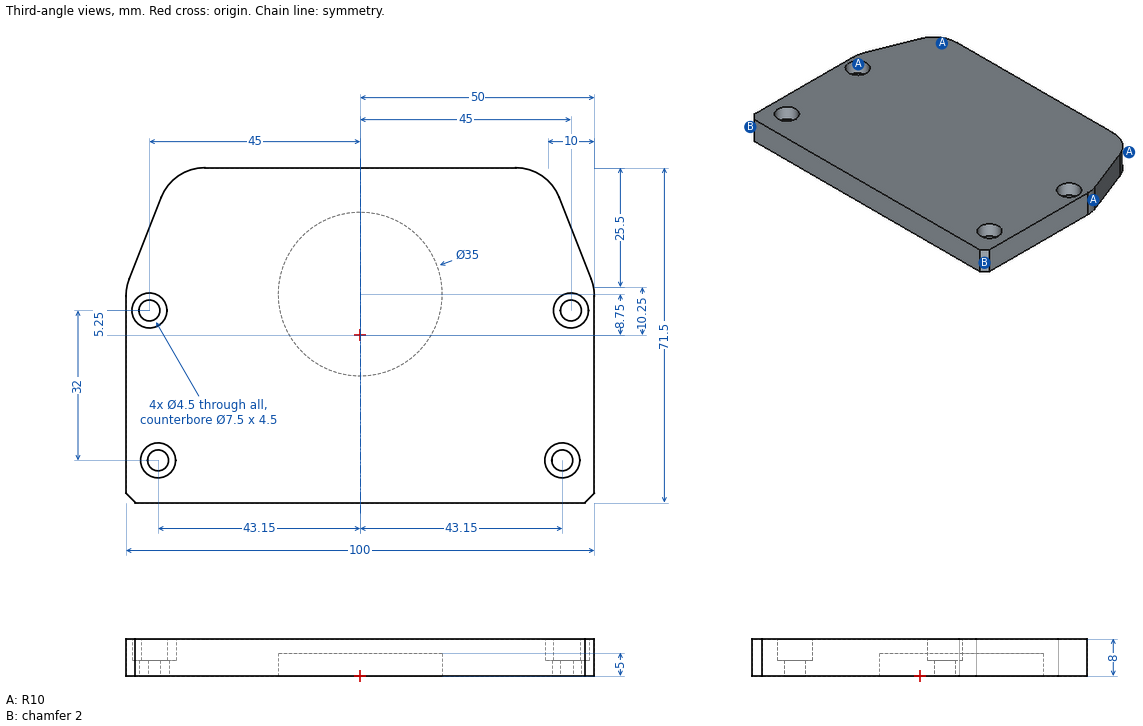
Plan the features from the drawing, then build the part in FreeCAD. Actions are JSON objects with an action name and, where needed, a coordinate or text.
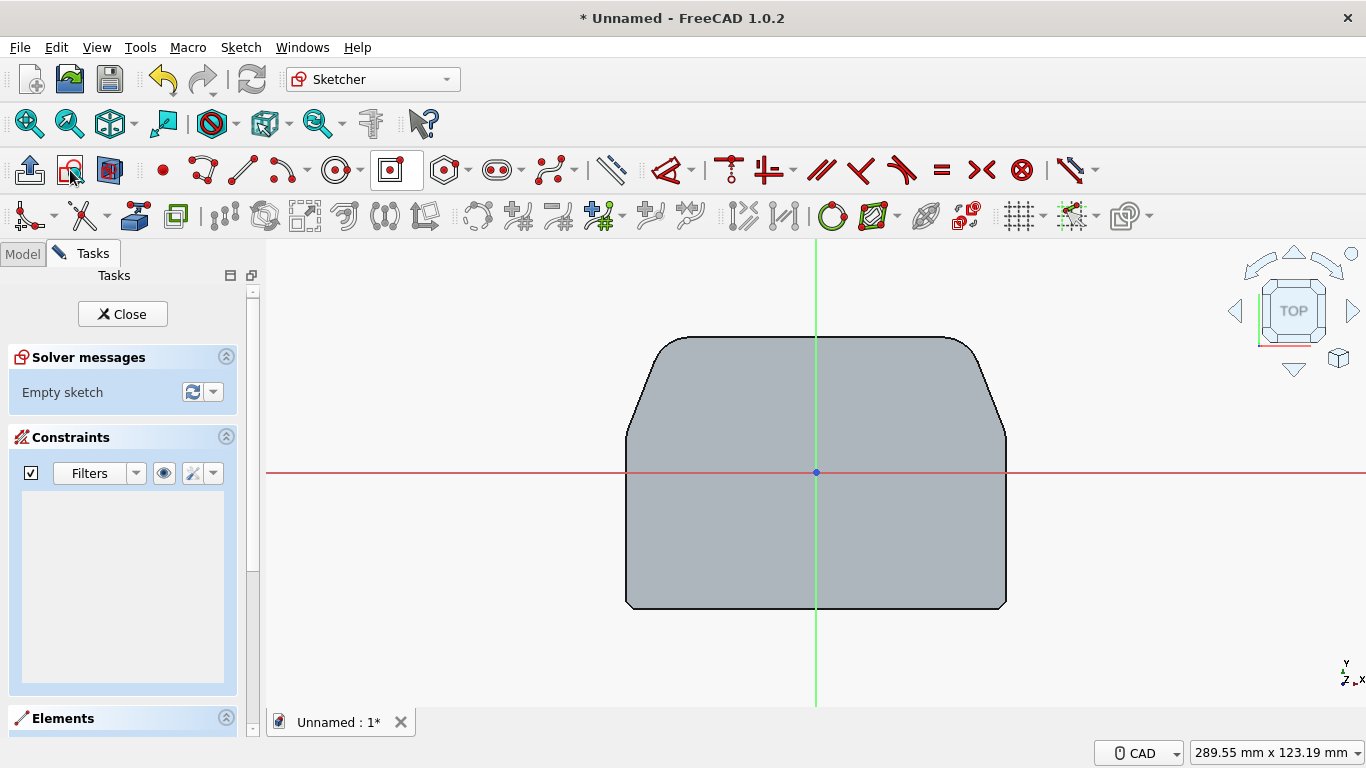
{"action": "scroll", "coordinate": [899, 564], "scroll_direction": "up", "scroll_amount": 3}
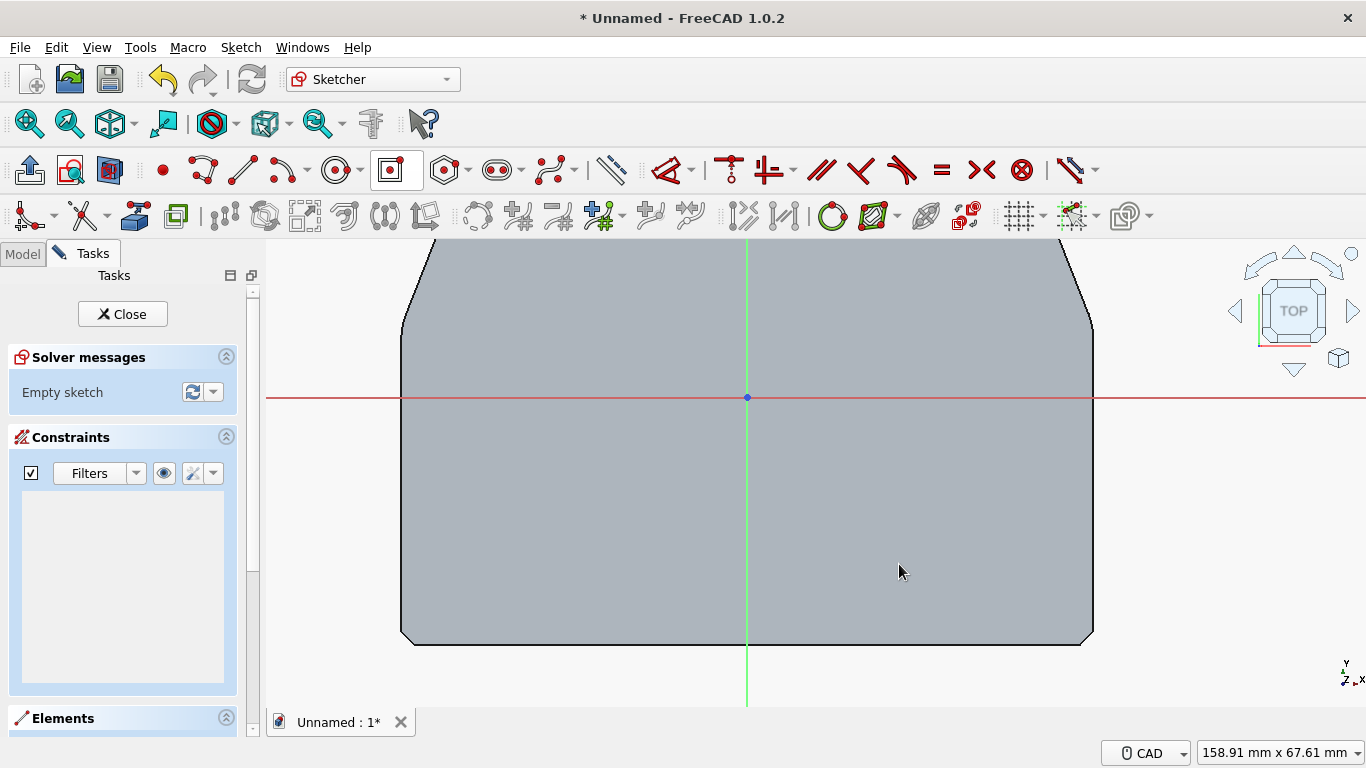
{"action": "left_click", "coordinate": [336, 170]}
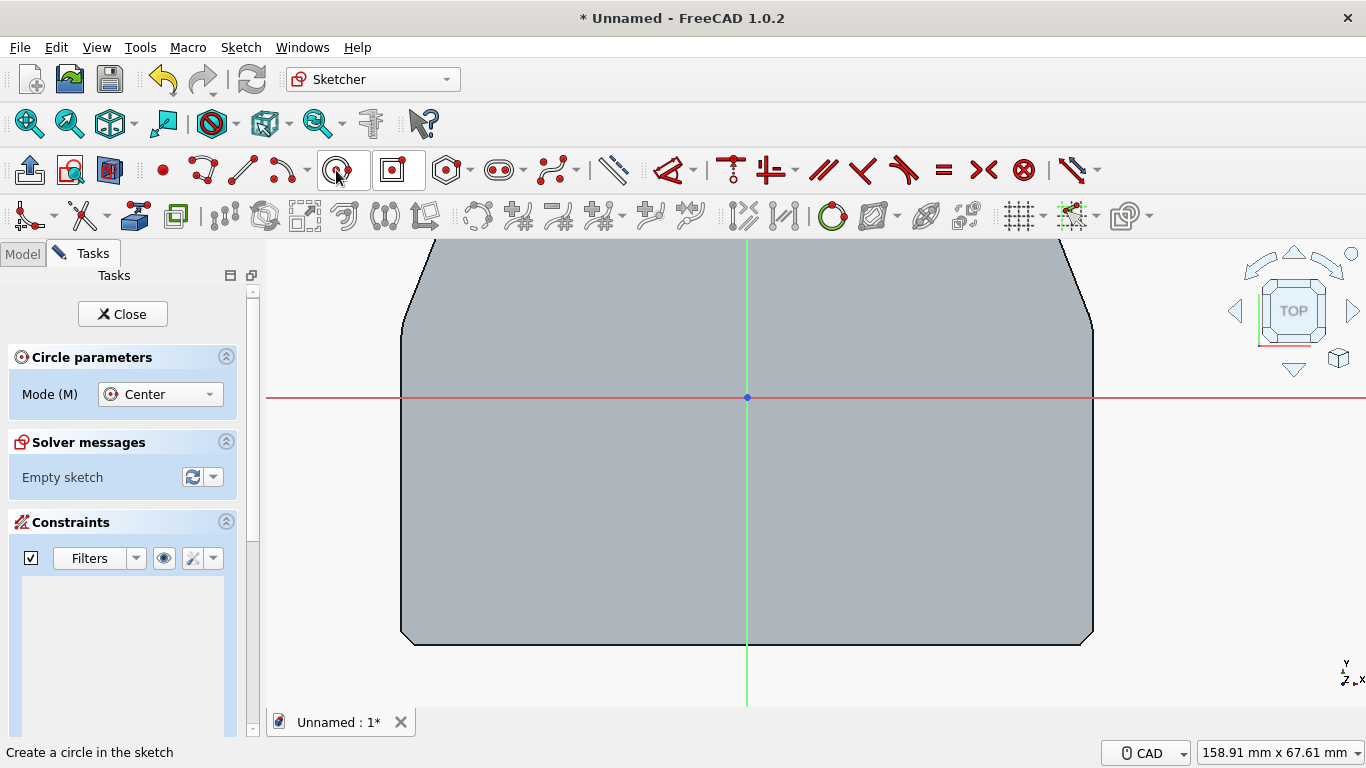
{"action": "scroll", "coordinate": [436, 361], "scroll_direction": "up", "scroll_amount": 2}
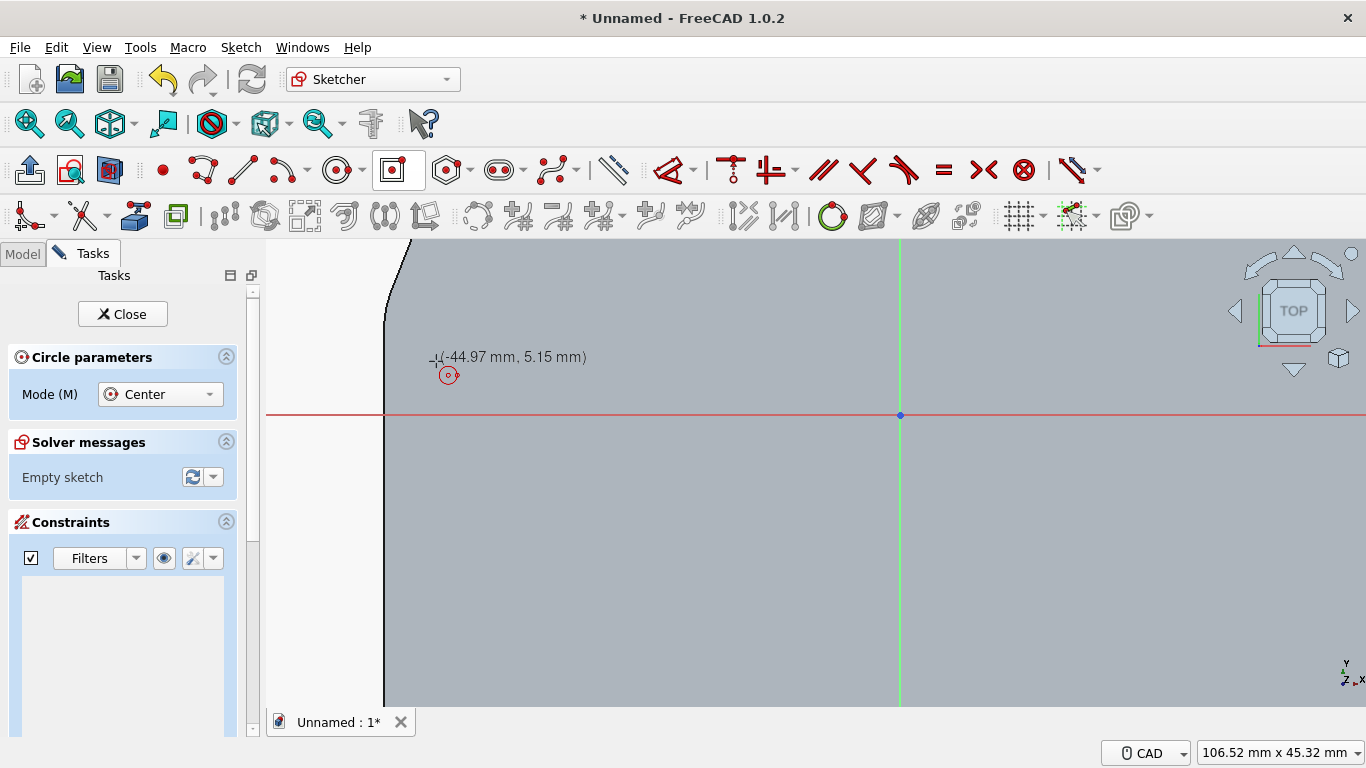
{"action": "left_click", "coordinate": [436, 361]}
{"action": "left_click", "coordinate": [452, 345]}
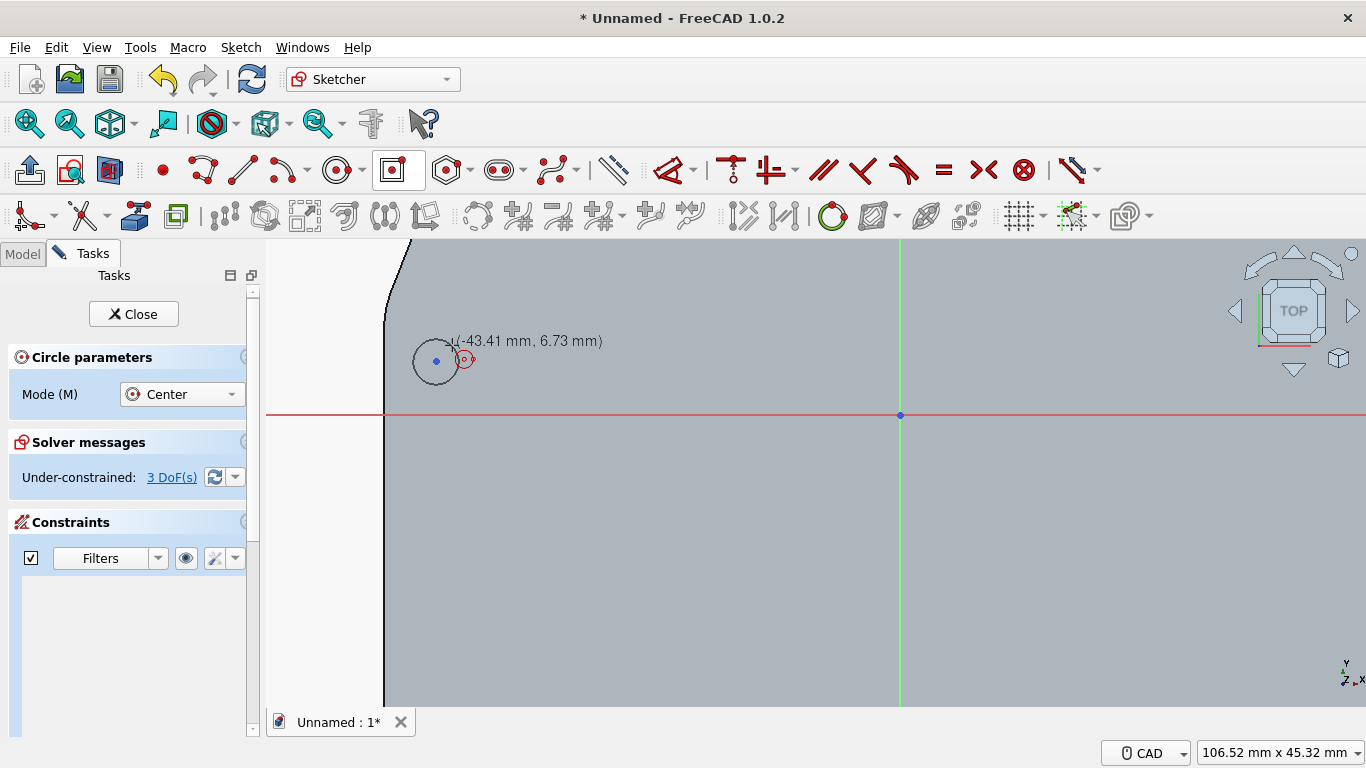
{"action": "scroll", "coordinate": [437, 364], "scroll_direction": "down", "scroll_amount": 2}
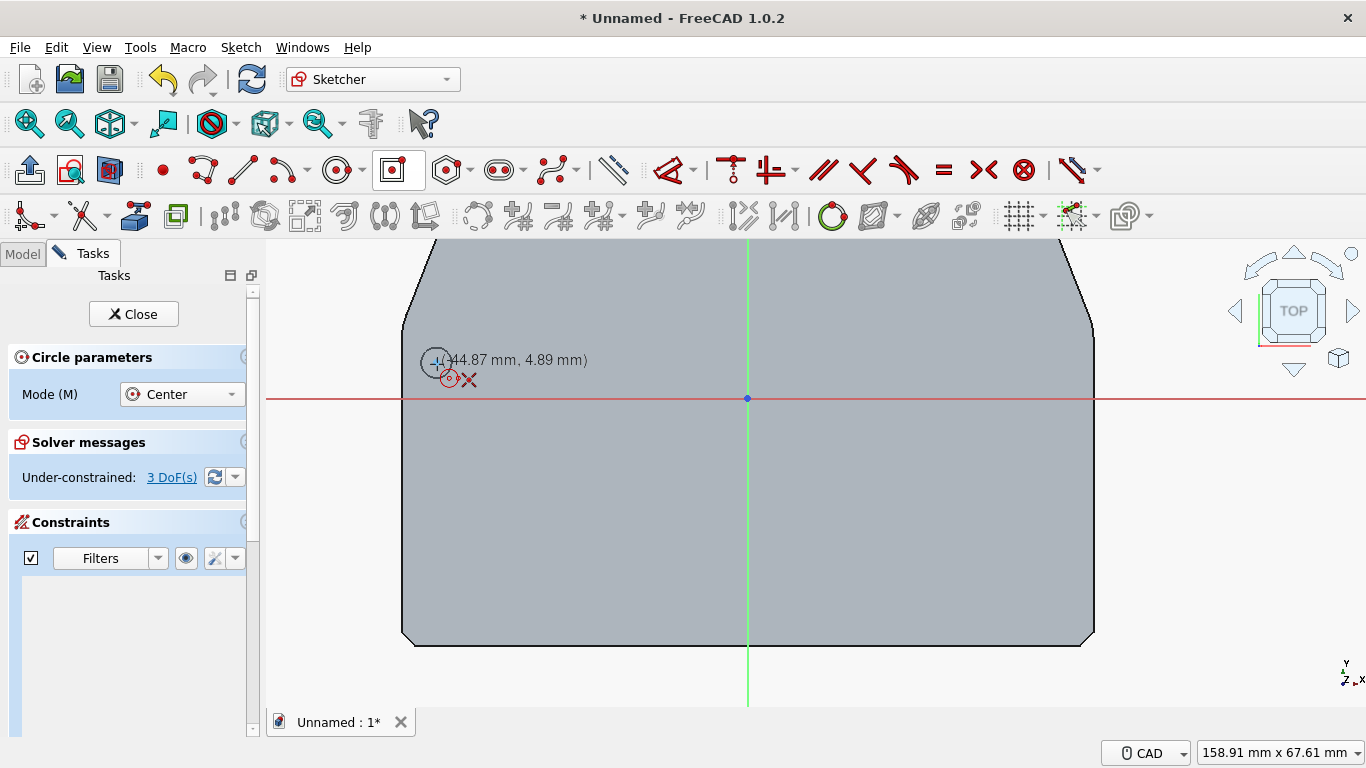
{"action": "scroll", "coordinate": [449, 584], "scroll_direction": "up", "scroll_amount": 2}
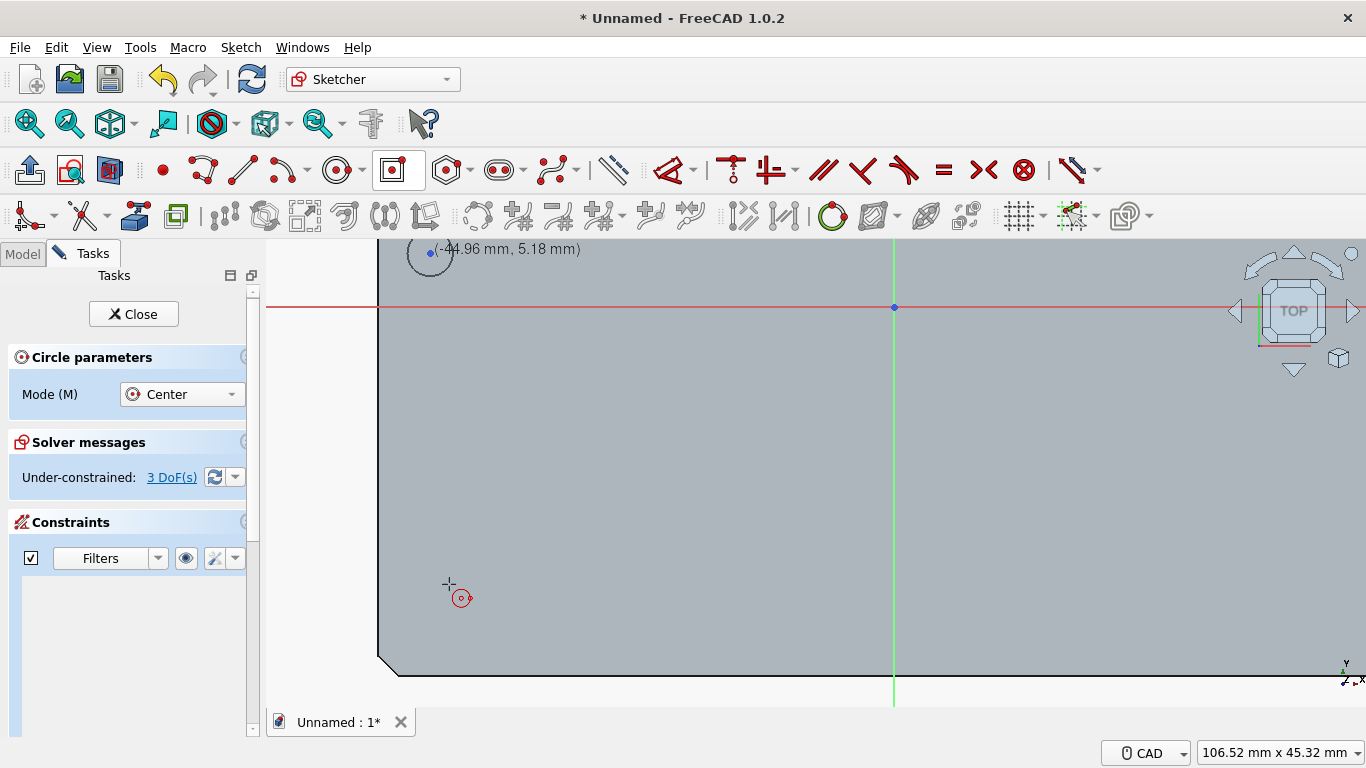
{"action": "left_click", "coordinate": [449, 583]}
{"action": "left_click", "coordinate": [465, 567]}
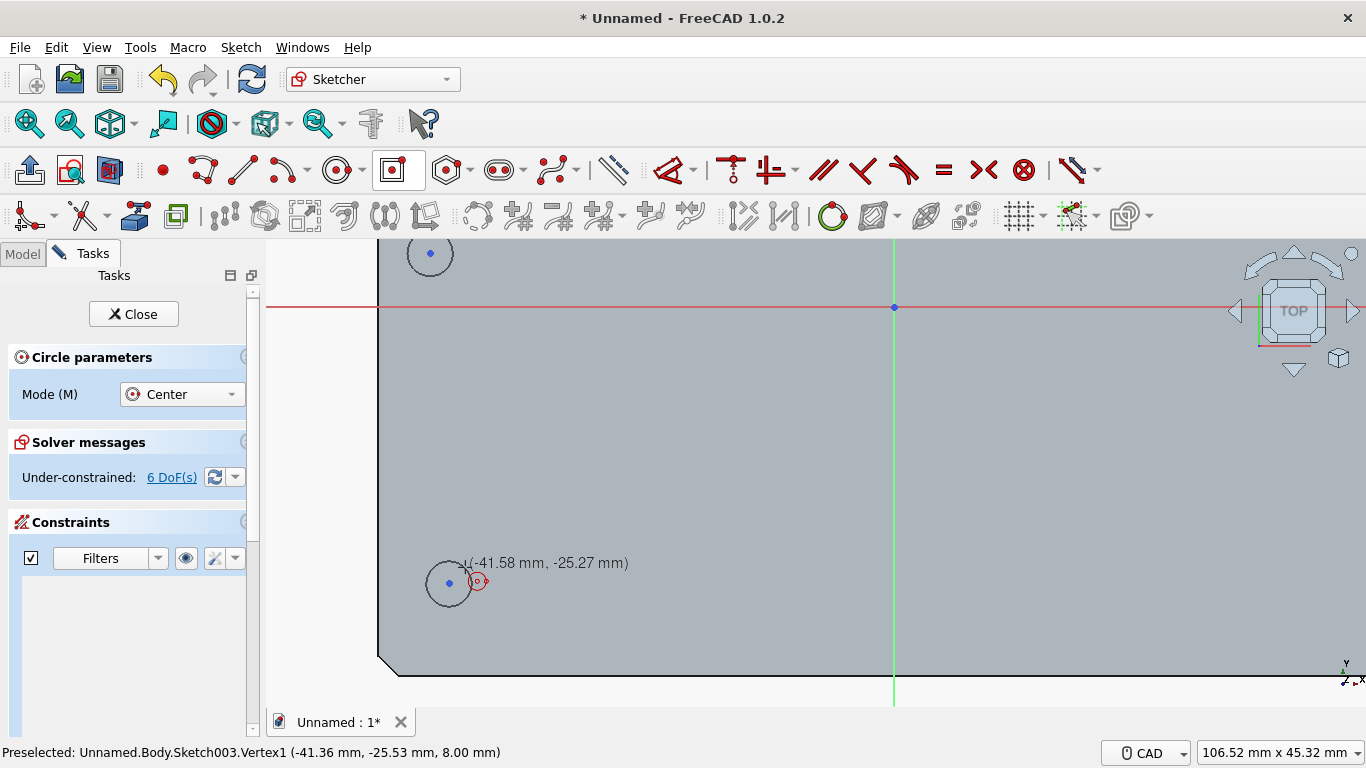
{"action": "scroll", "coordinate": [449, 585], "scroll_direction": "down", "scroll_amount": 2}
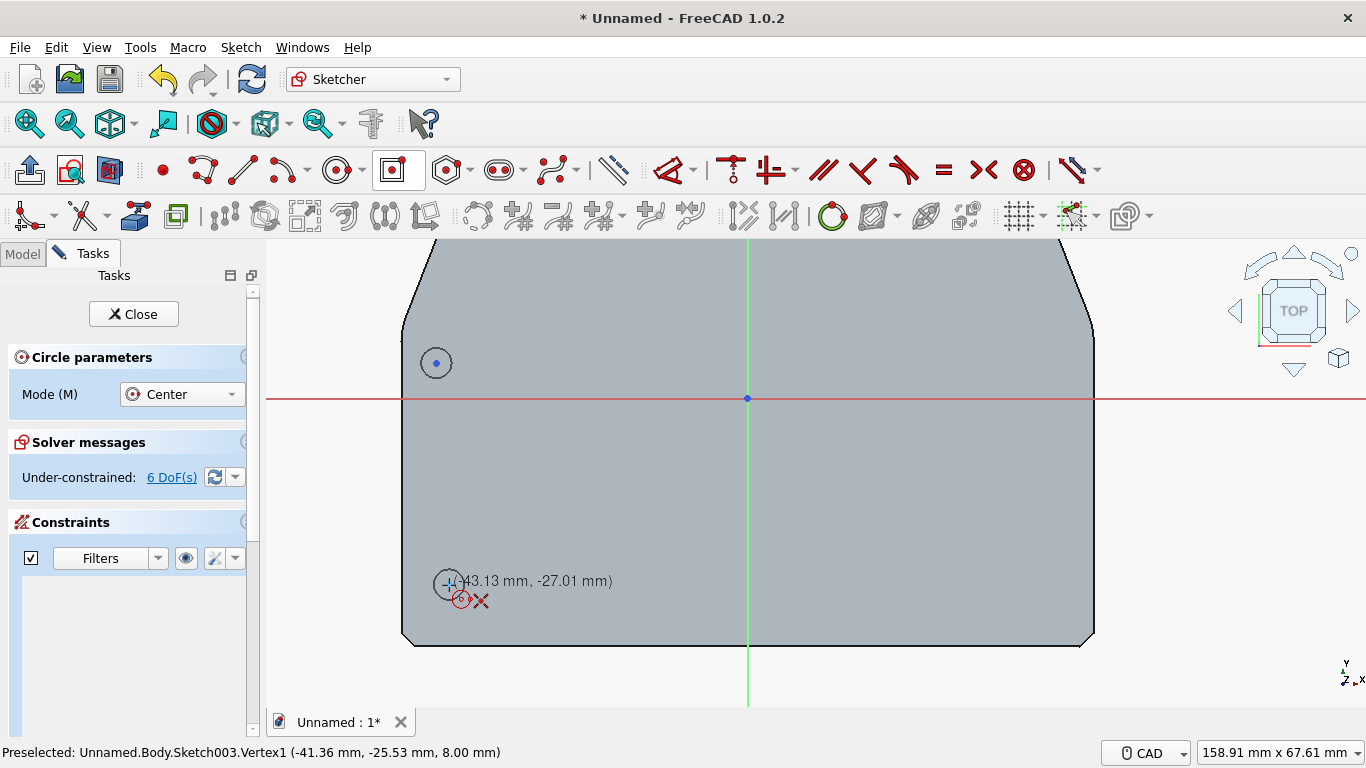
{"action": "scroll", "coordinate": [1059, 363], "scroll_direction": "up", "scroll_amount": 2}